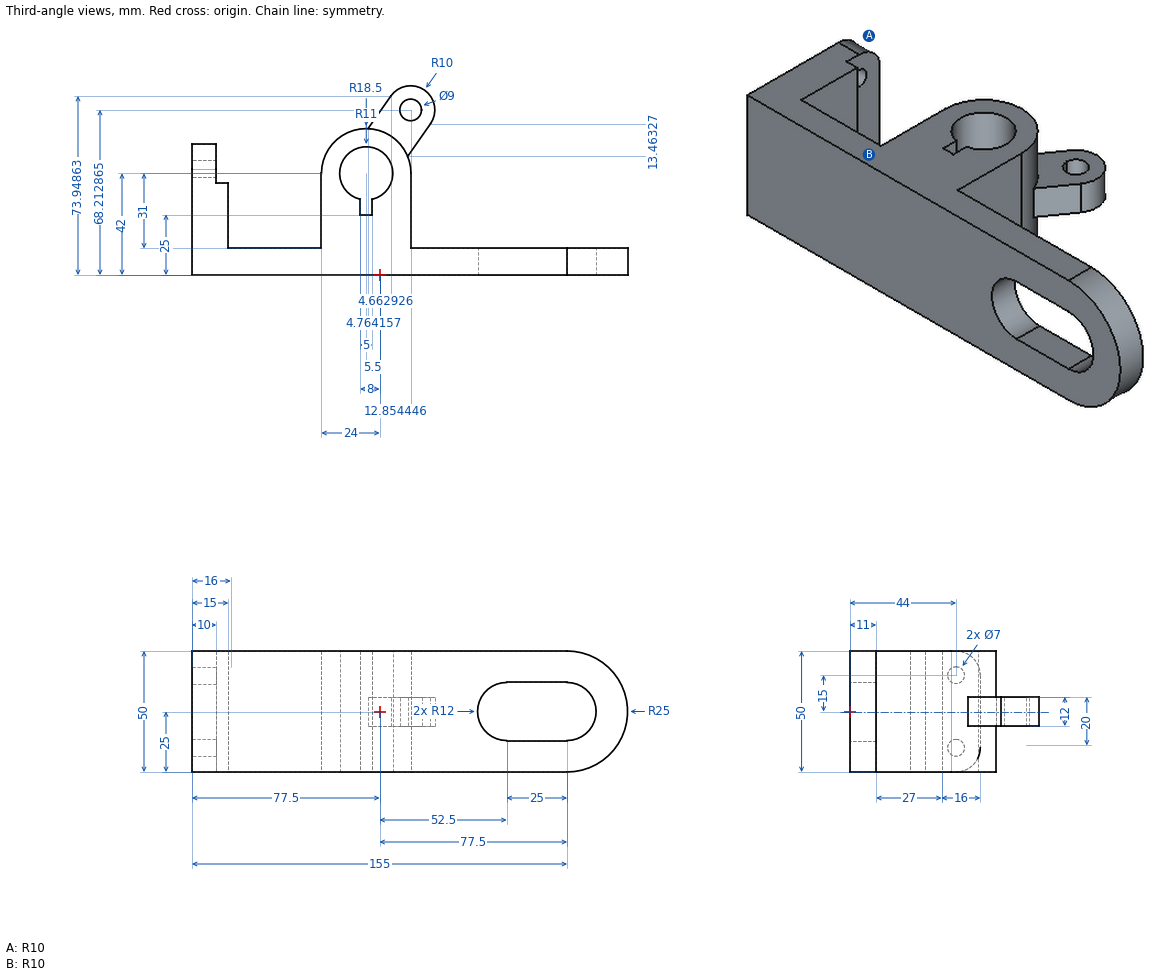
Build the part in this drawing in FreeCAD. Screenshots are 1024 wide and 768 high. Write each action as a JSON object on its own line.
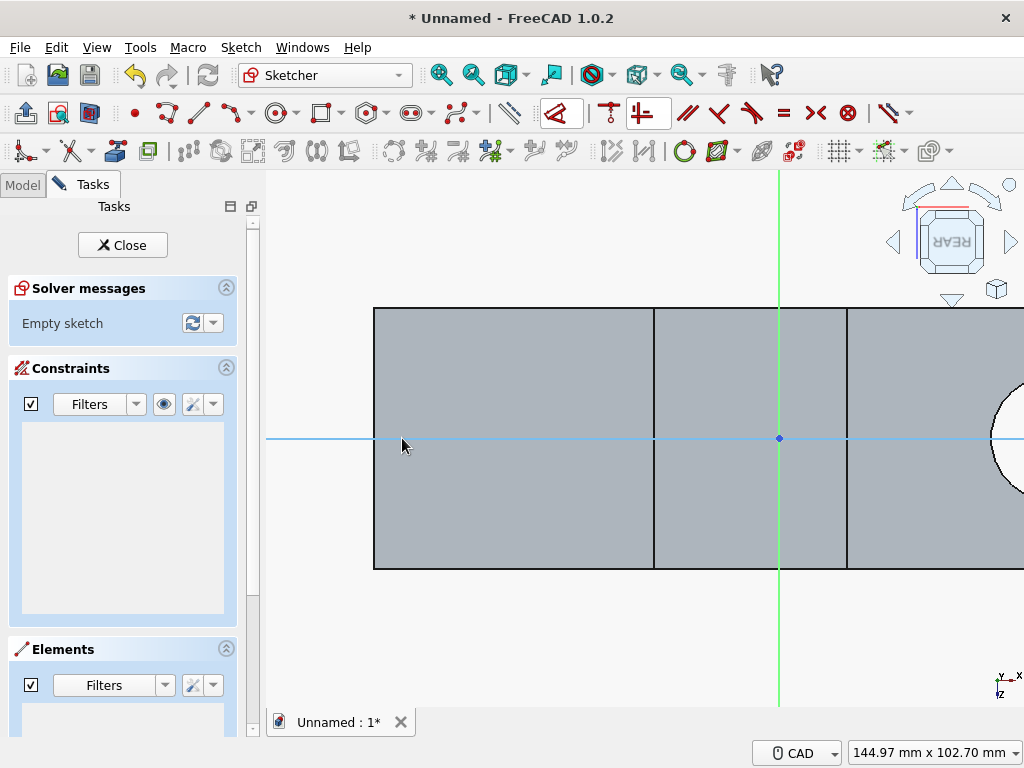
{"action": "left_click", "coordinate": [322, 114]}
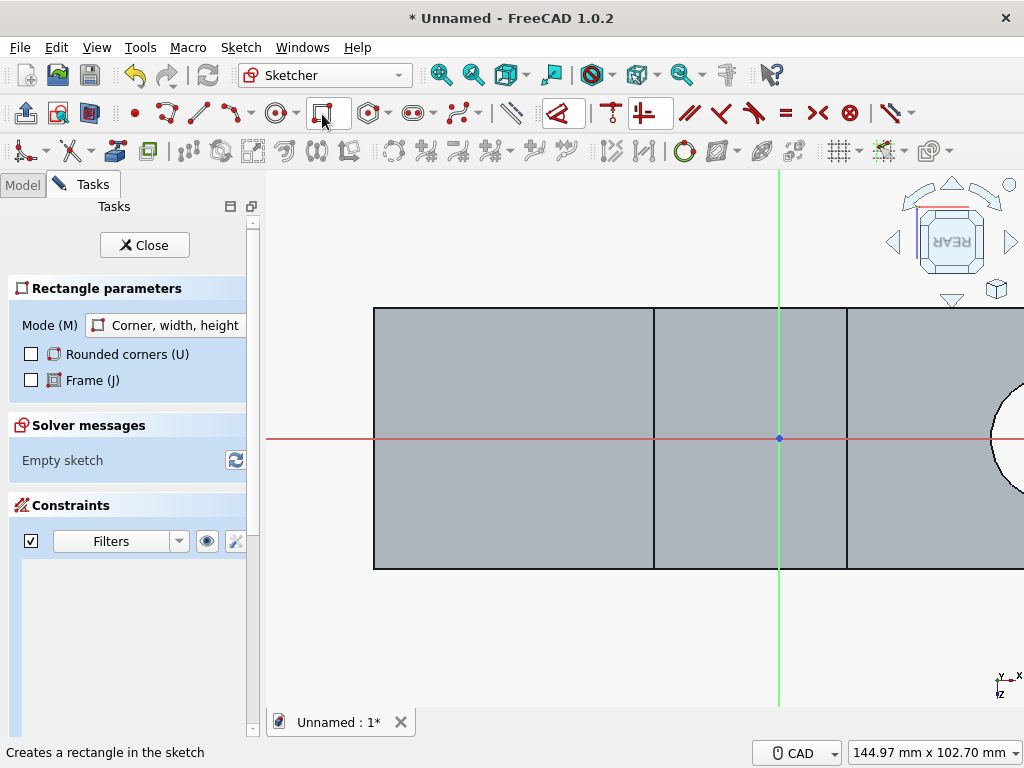
{"action": "left_click", "coordinate": [374, 308]}
{"action": "left_click", "coordinate": [452, 569]}
{"action": "key", "text": "Escape"}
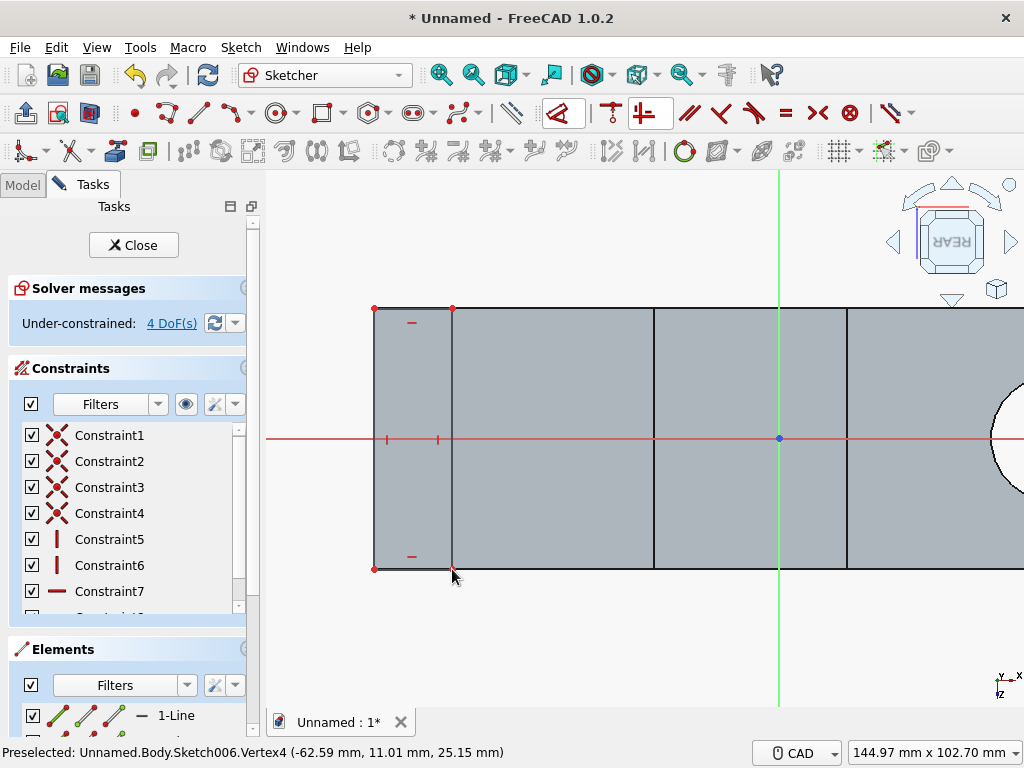
{"action": "left_click", "coordinate": [374, 387]}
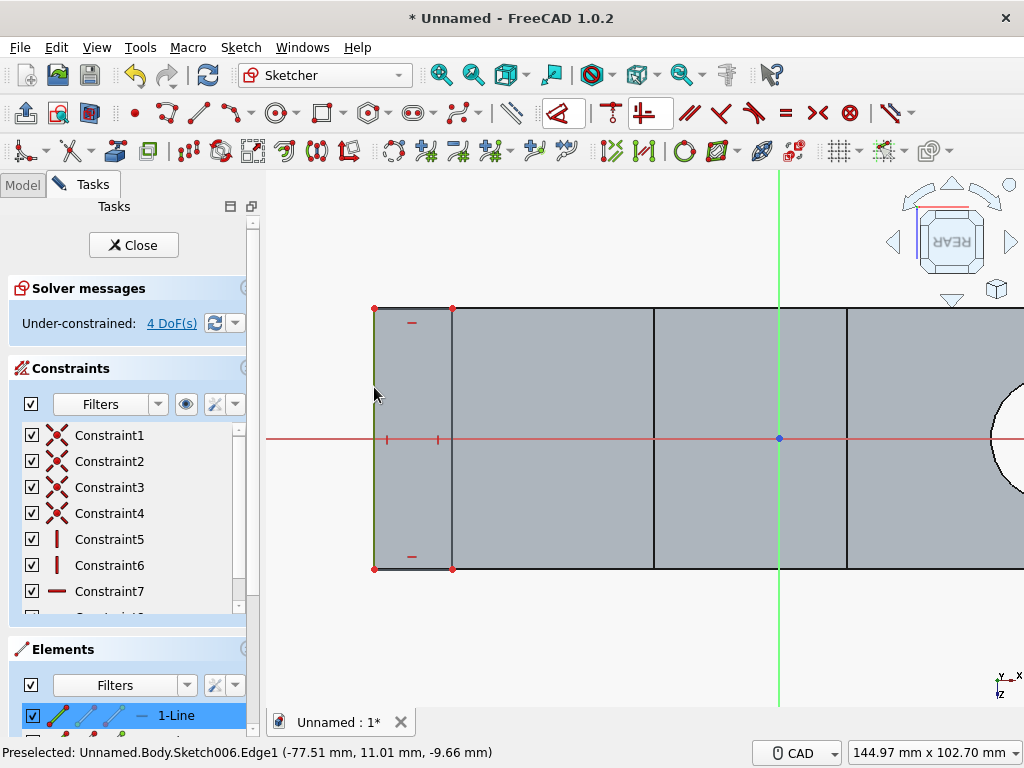
{"action": "key", "text": "i"}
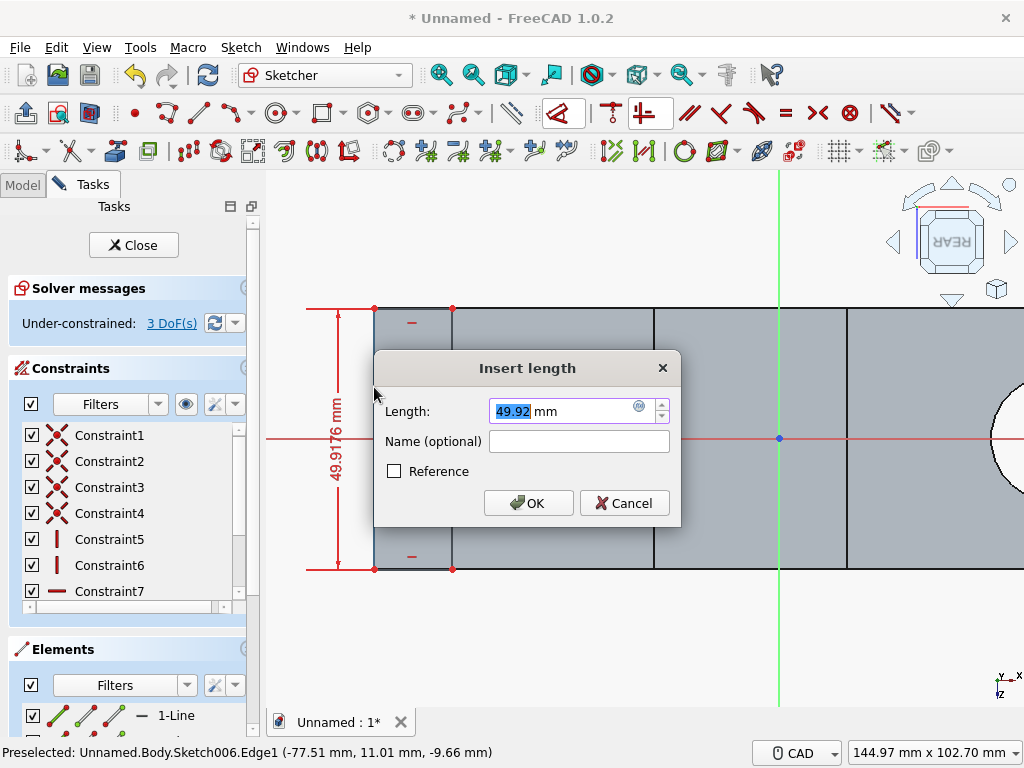
{"action": "type", "text": "50"}
{"action": "key", "text": "Return"}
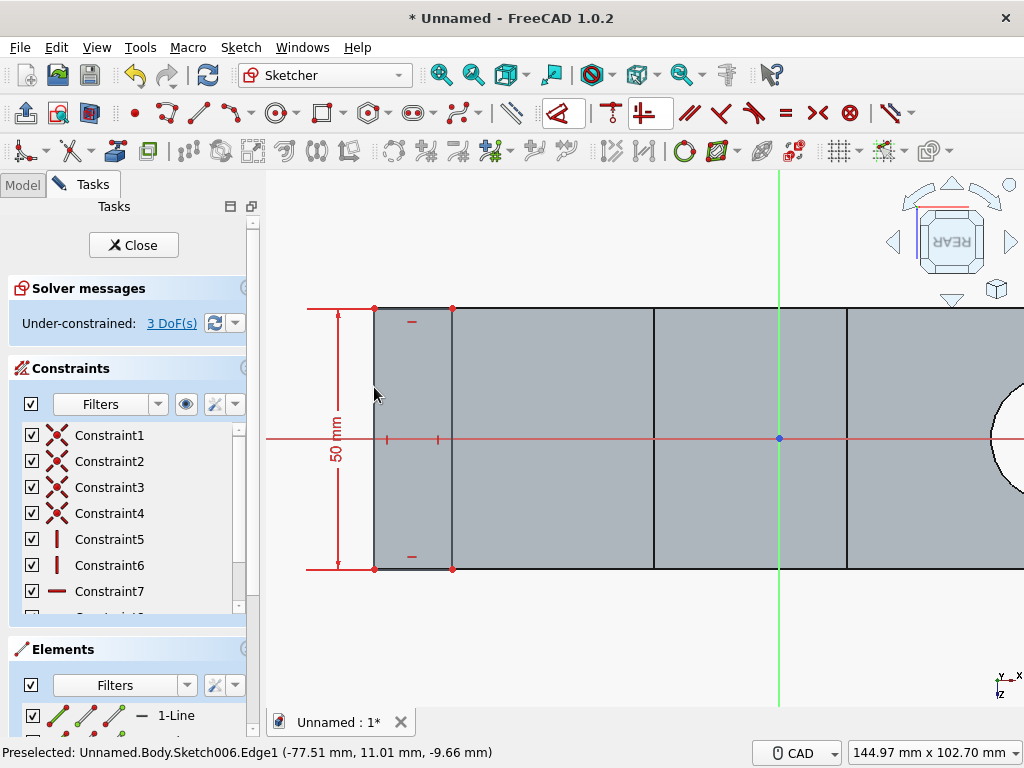
{"action": "left_click", "coordinate": [397, 570]}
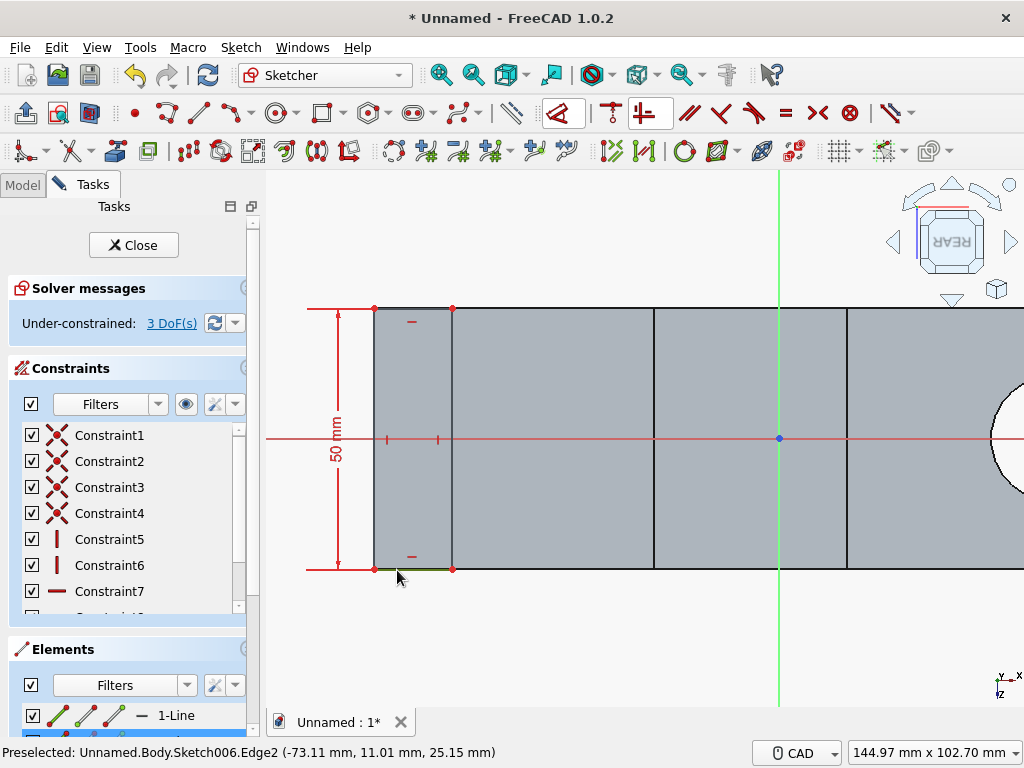
{"action": "key", "text": "l"}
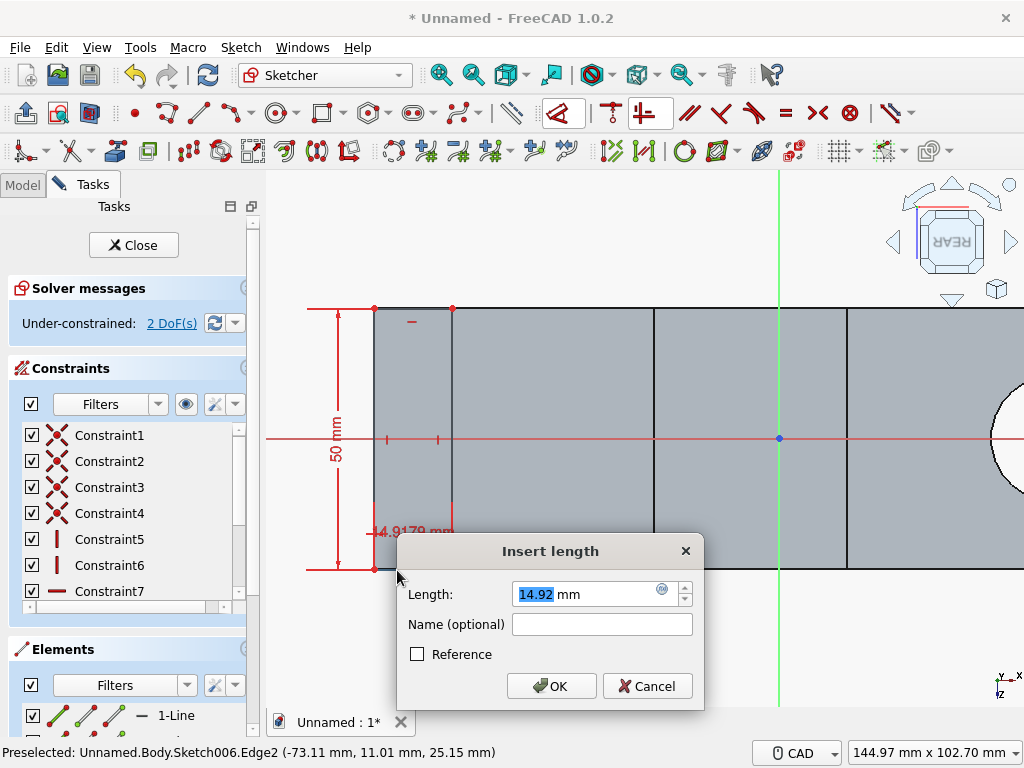
{"action": "type", "text": "15"}
{"action": "key", "text": "Return"}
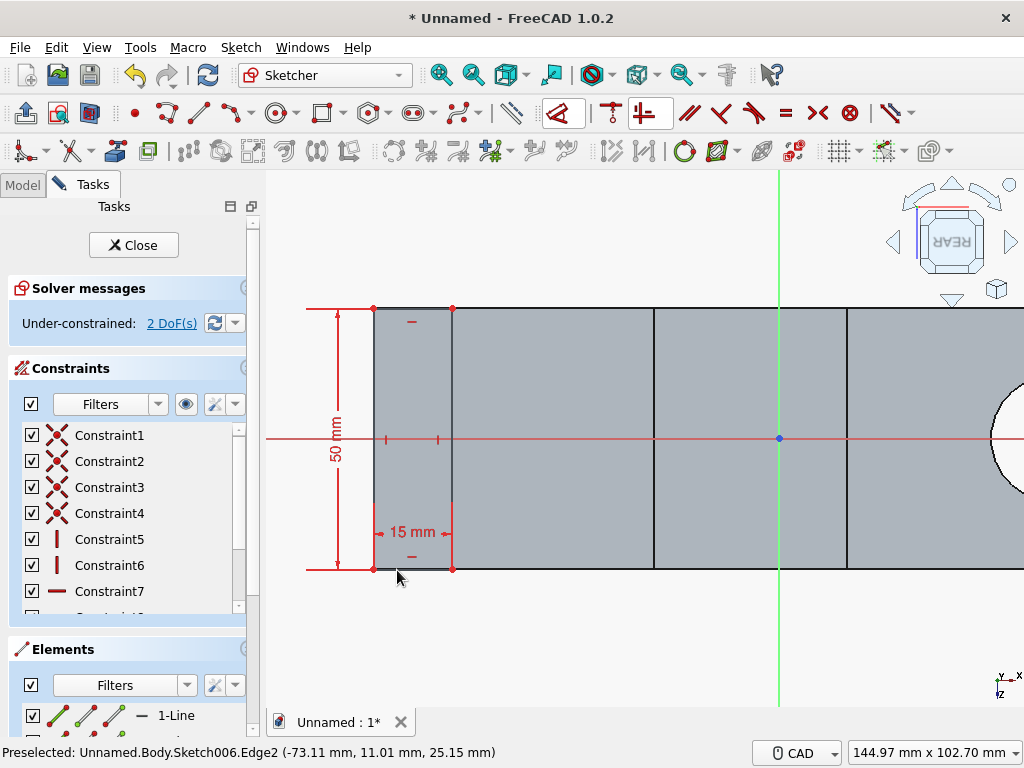
{"action": "left_click", "coordinate": [374, 309]}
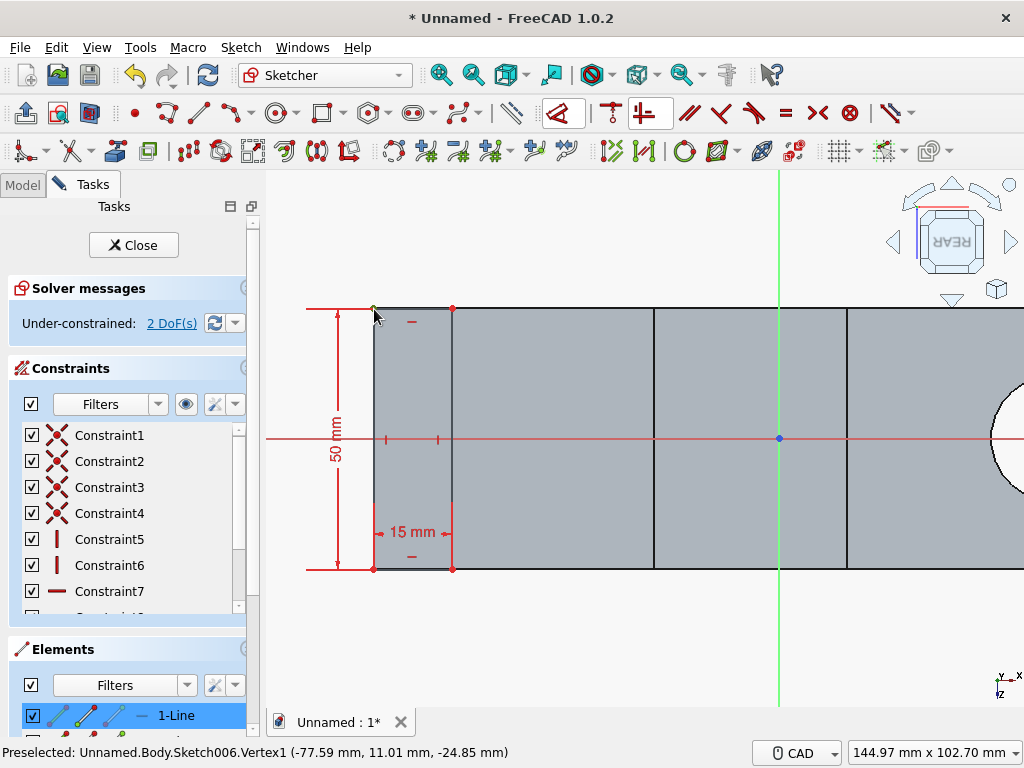
{"action": "left_click", "coordinate": [580, 114]}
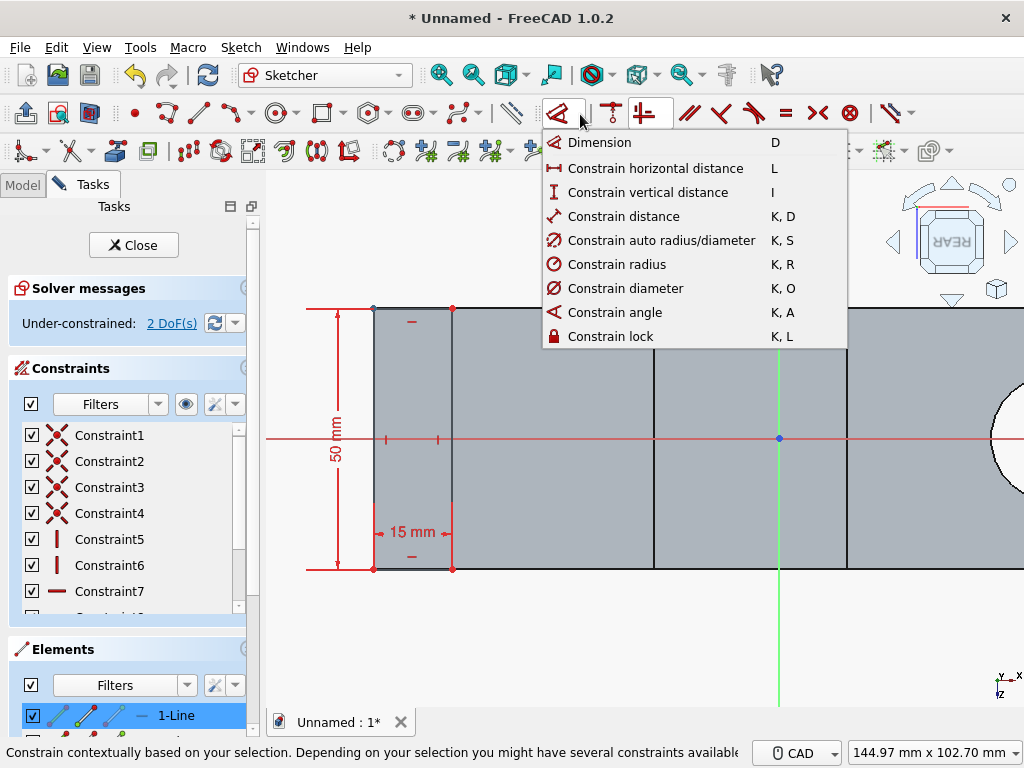
{"action": "left_click", "coordinate": [695, 192]}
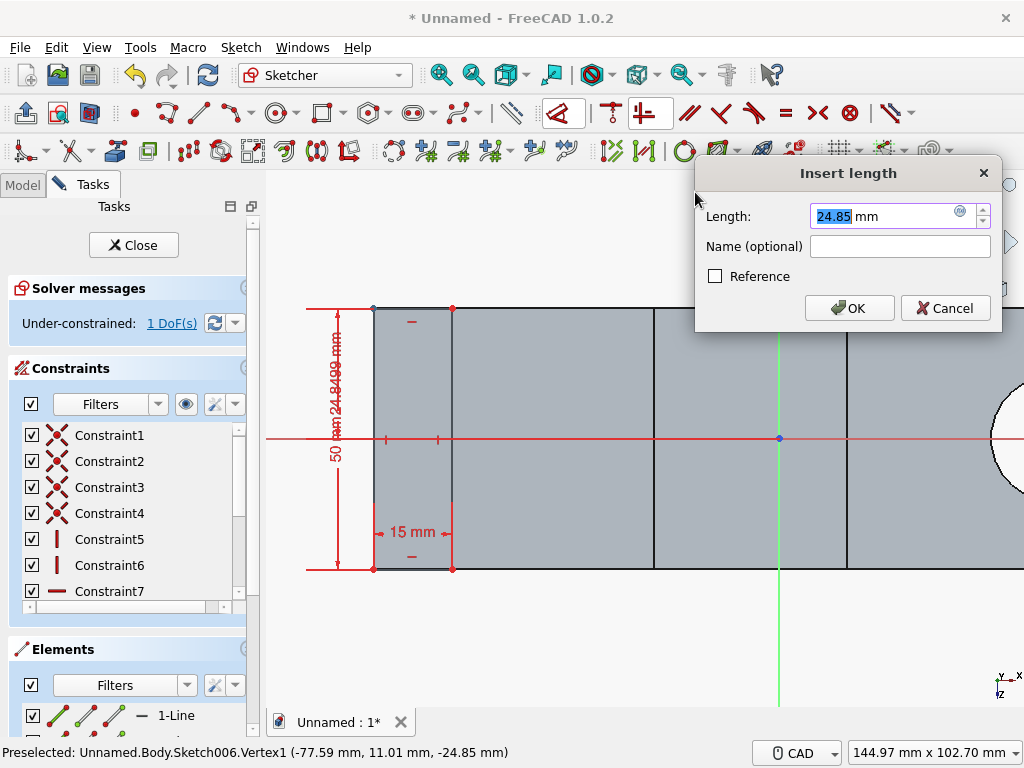
{"action": "type", "text": "25"}
{"action": "key", "text": "Return"}